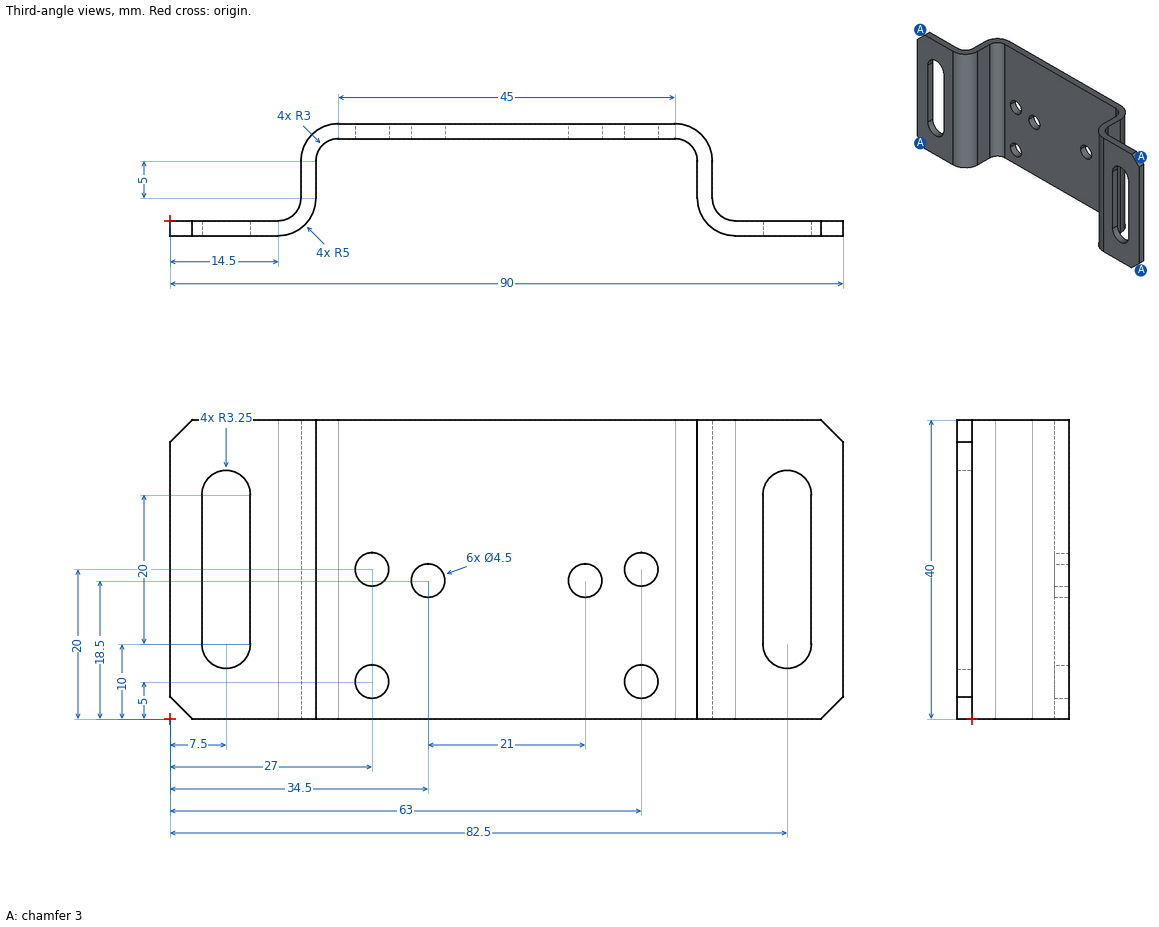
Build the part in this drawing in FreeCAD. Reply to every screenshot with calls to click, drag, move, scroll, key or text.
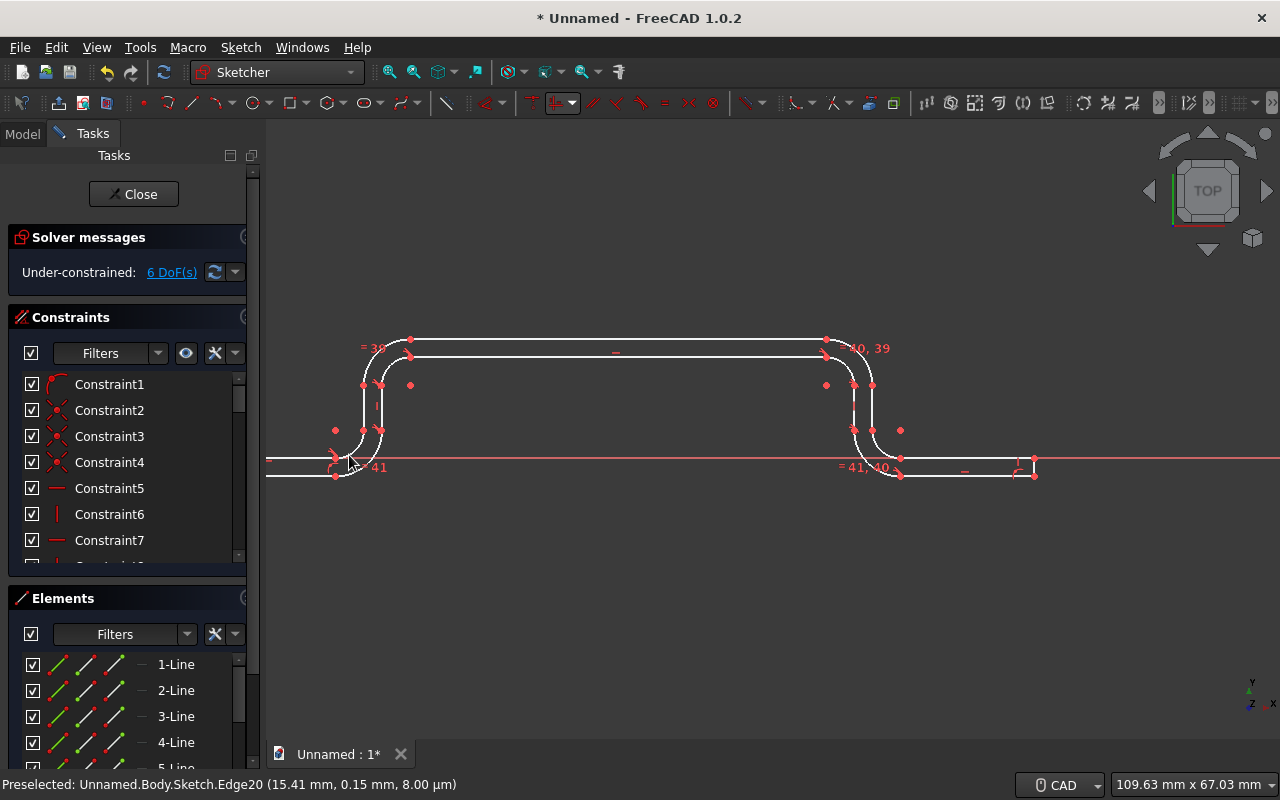
key(d)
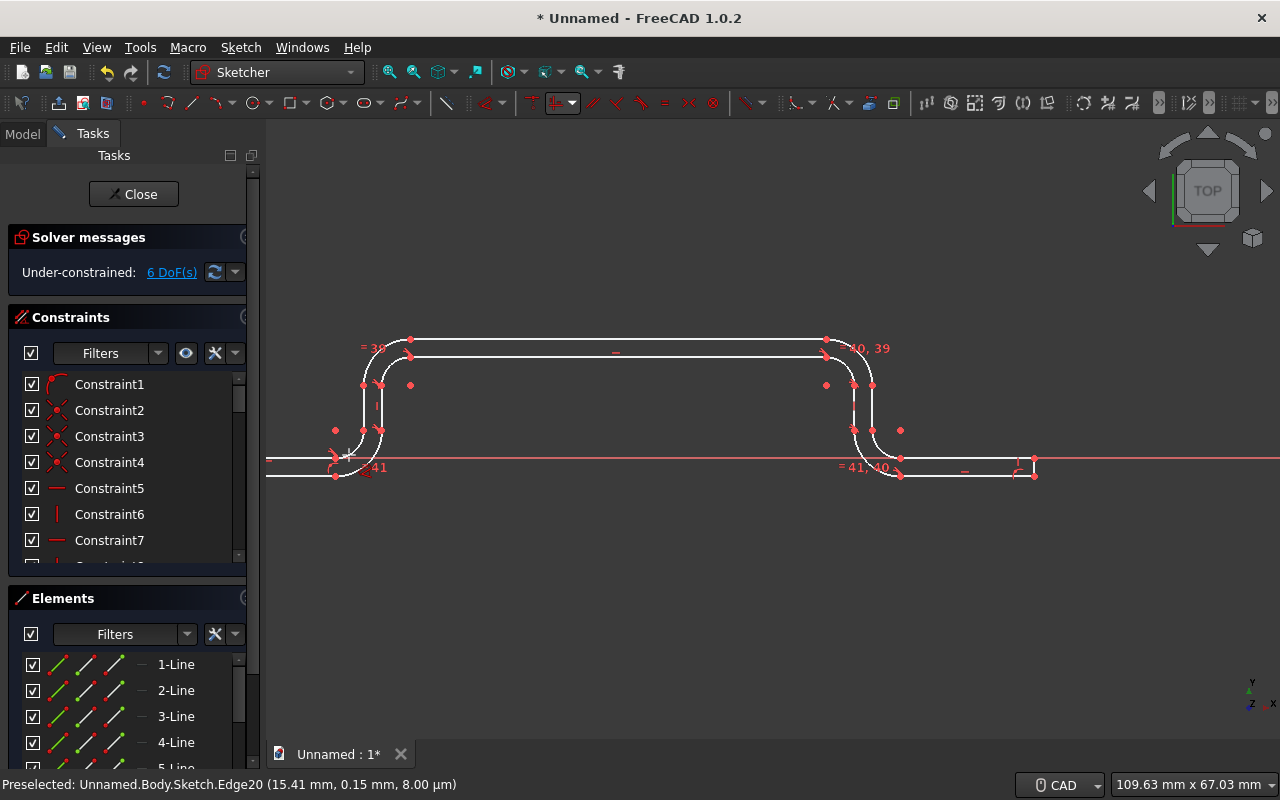
click(357, 471)
click(372, 499)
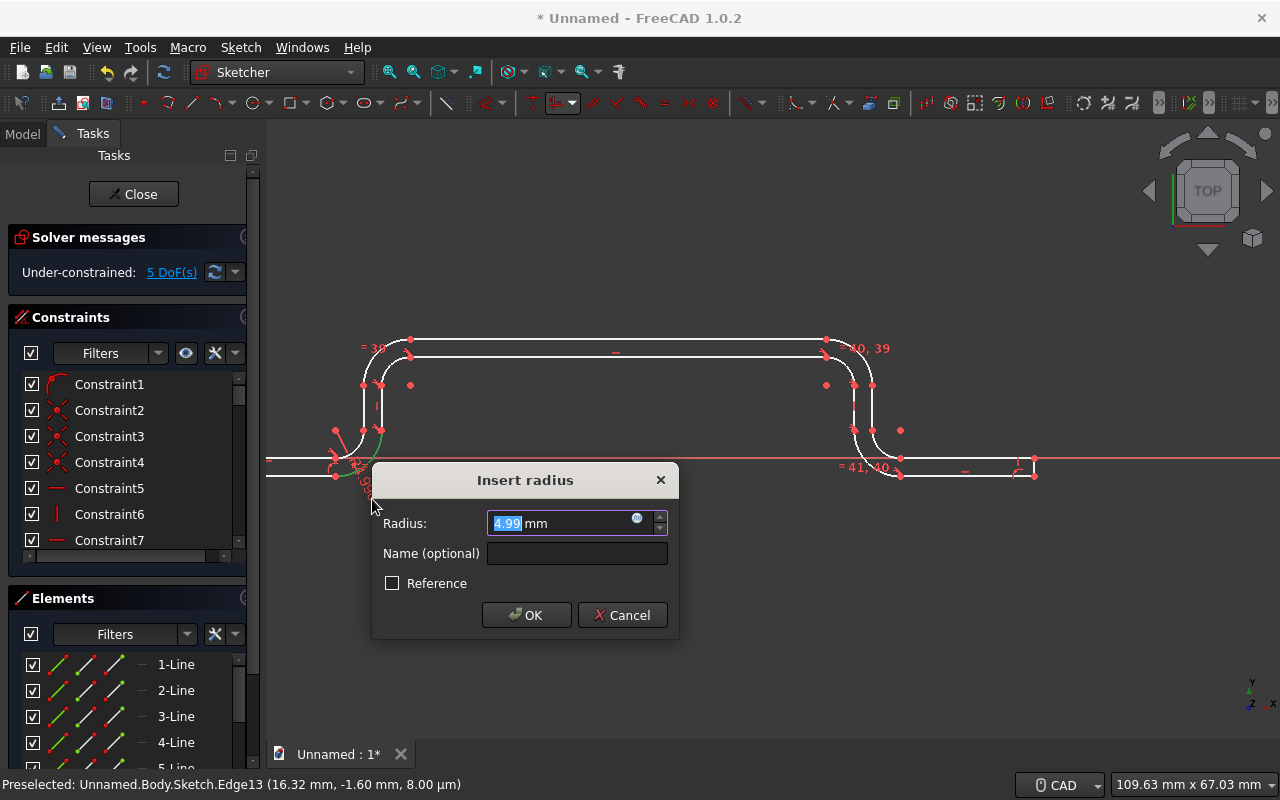
text(5)
key(Return)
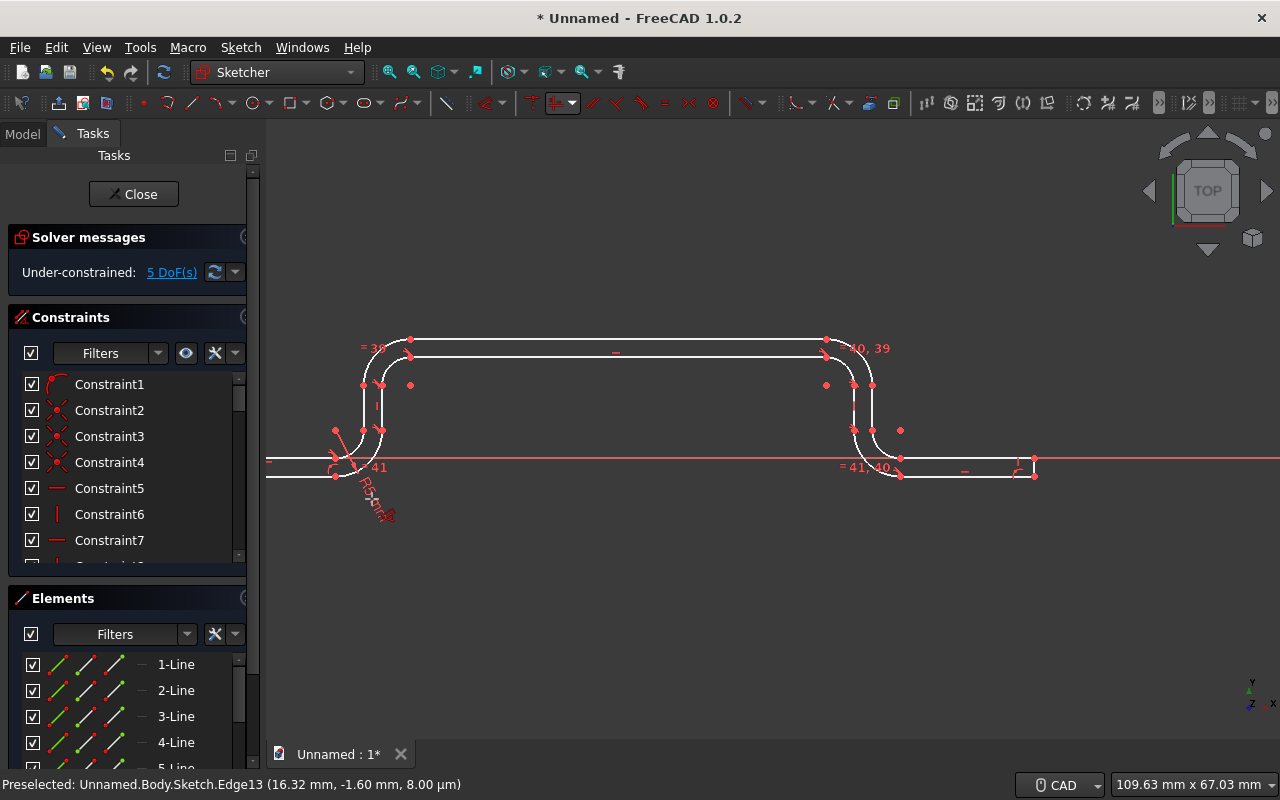
scroll(397, 361, up, 2)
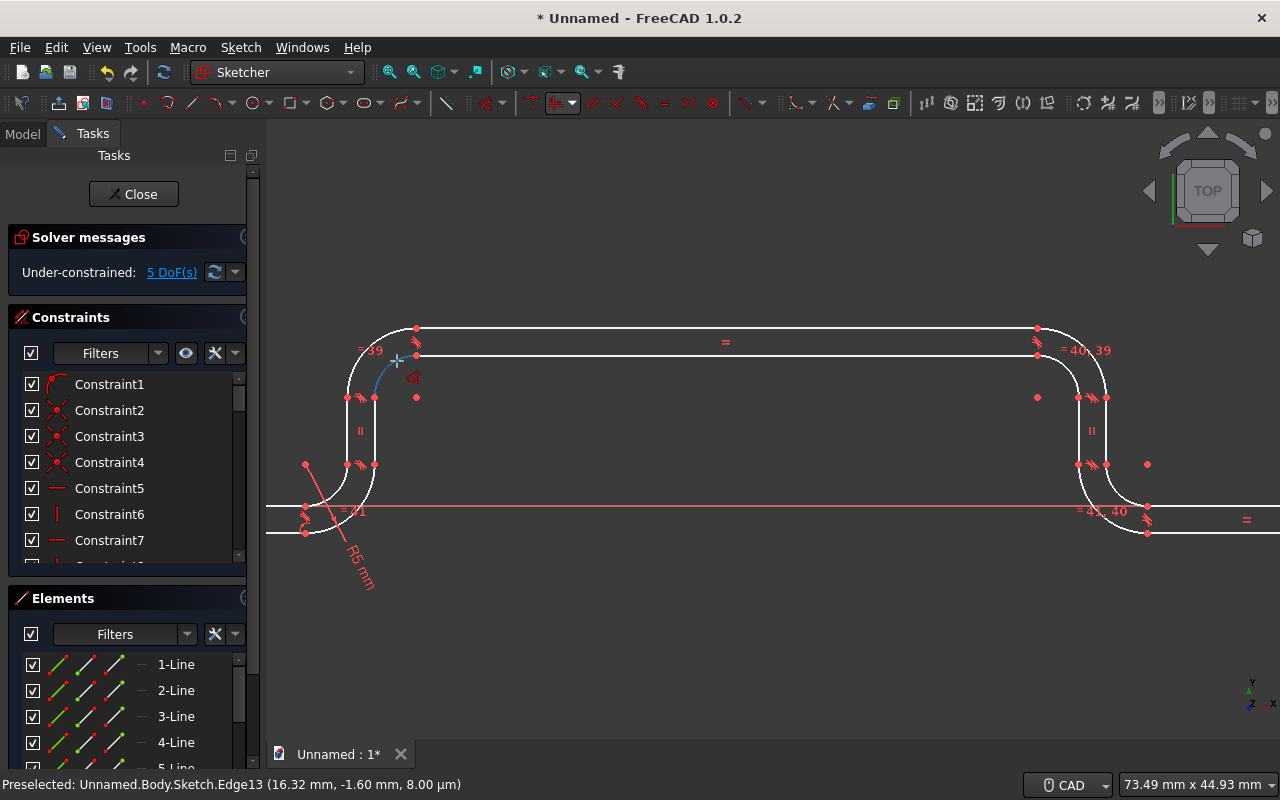
click(398, 360)
click(449, 463)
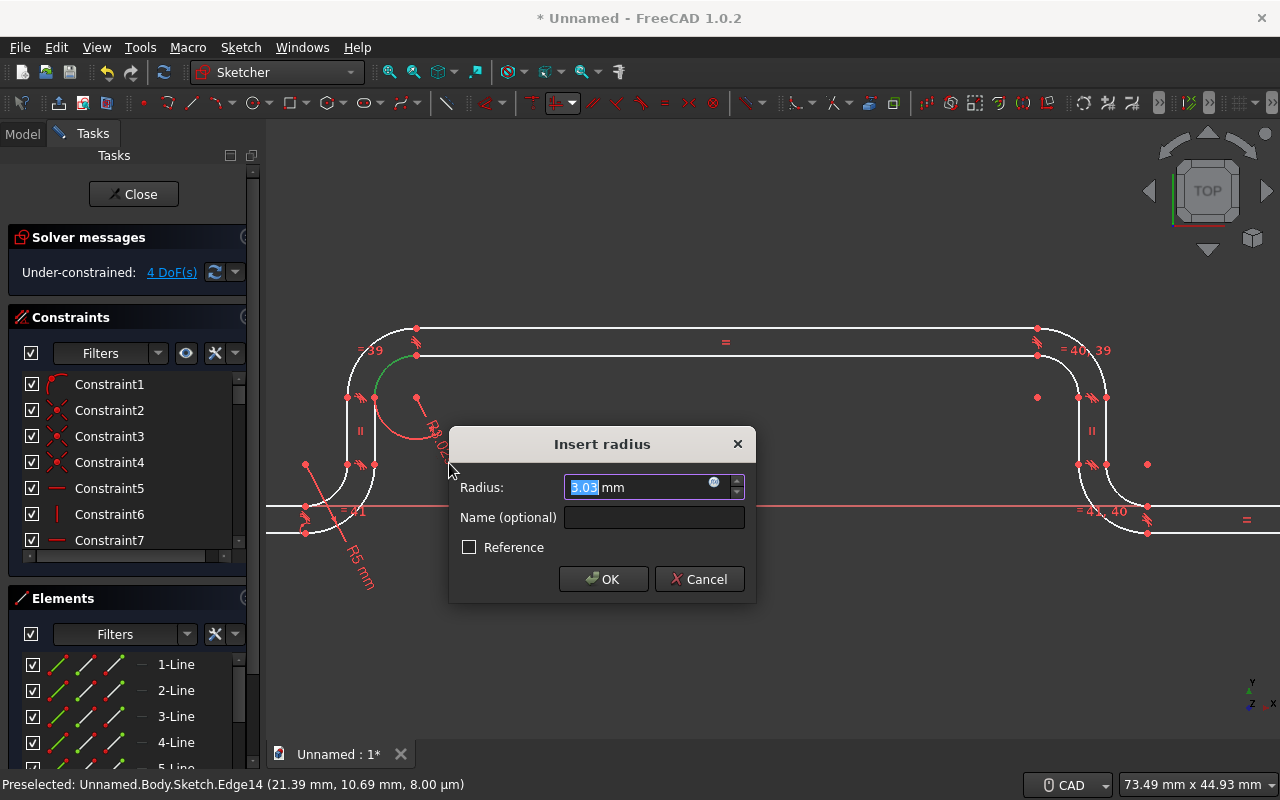
text(3)
key(Return)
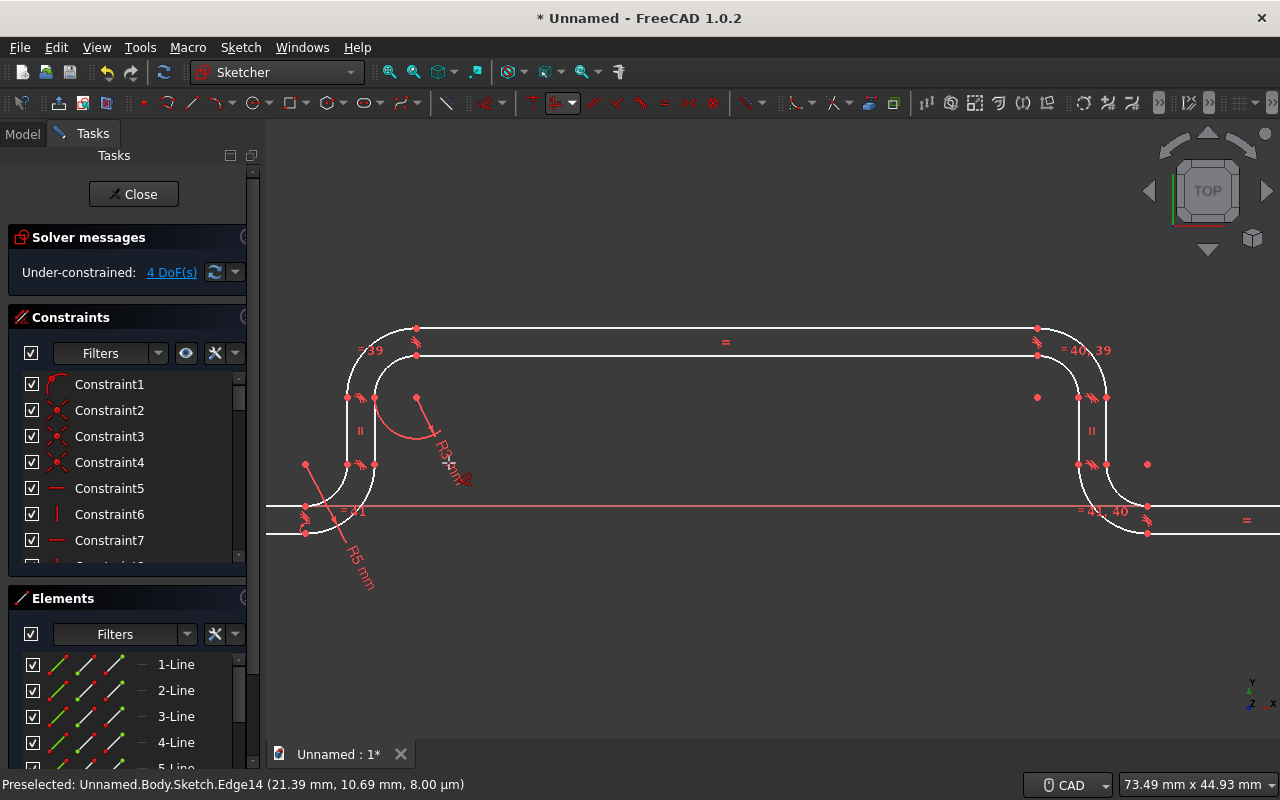
click(375, 444)
click(409, 431)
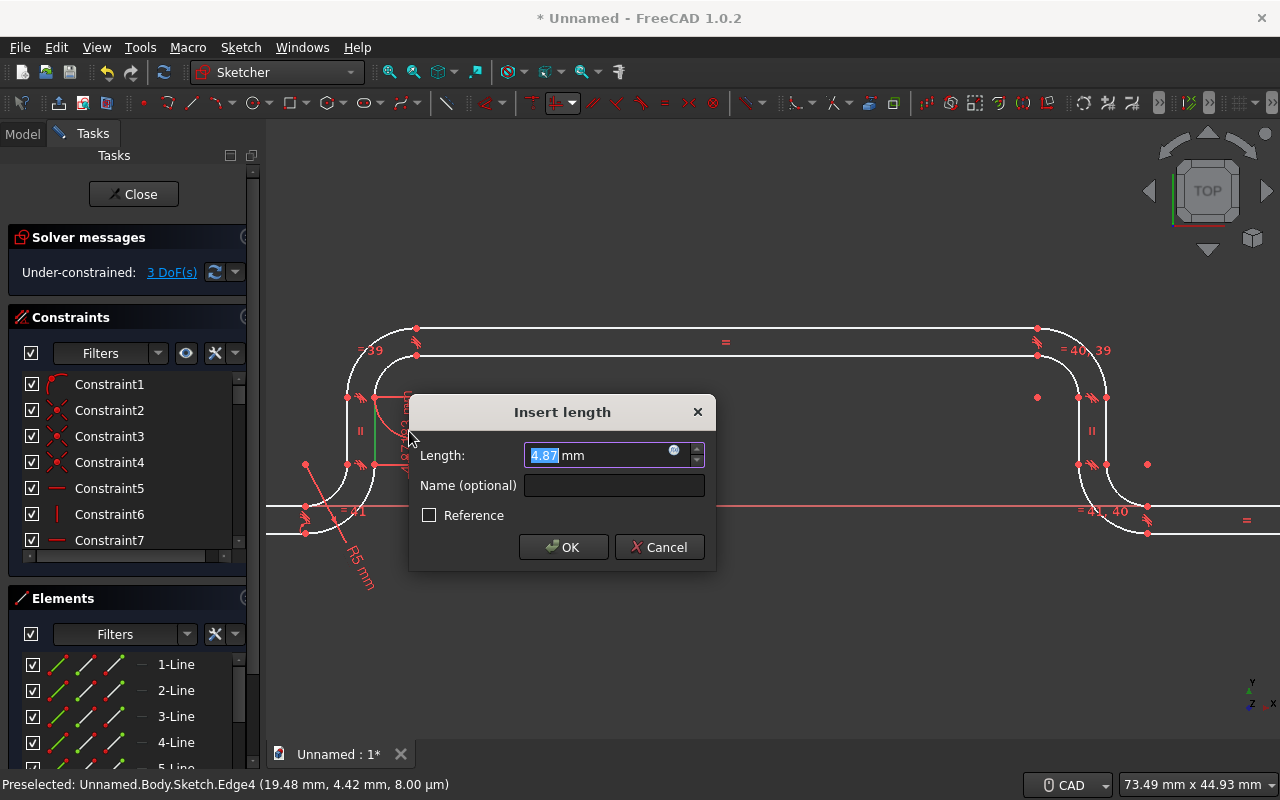
text(5)
key(Return)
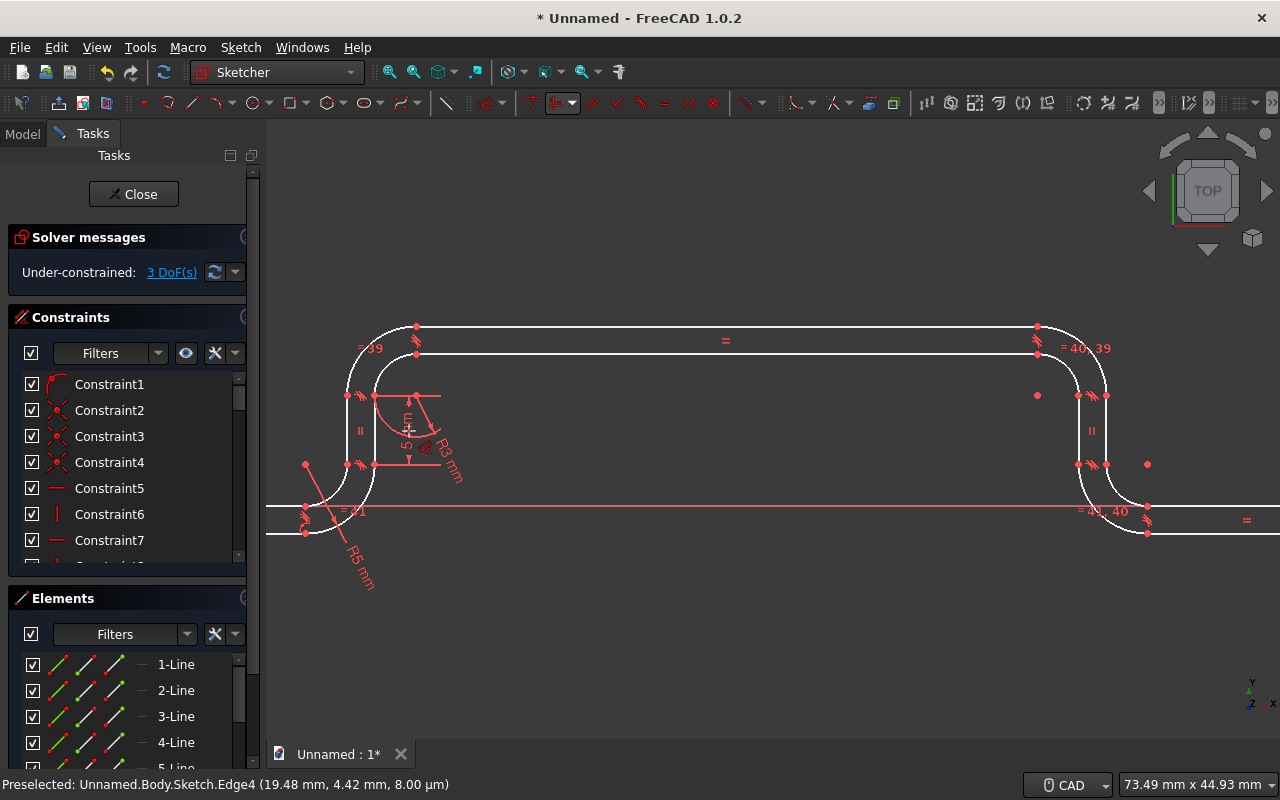
click(602, 354)
click(727, 388)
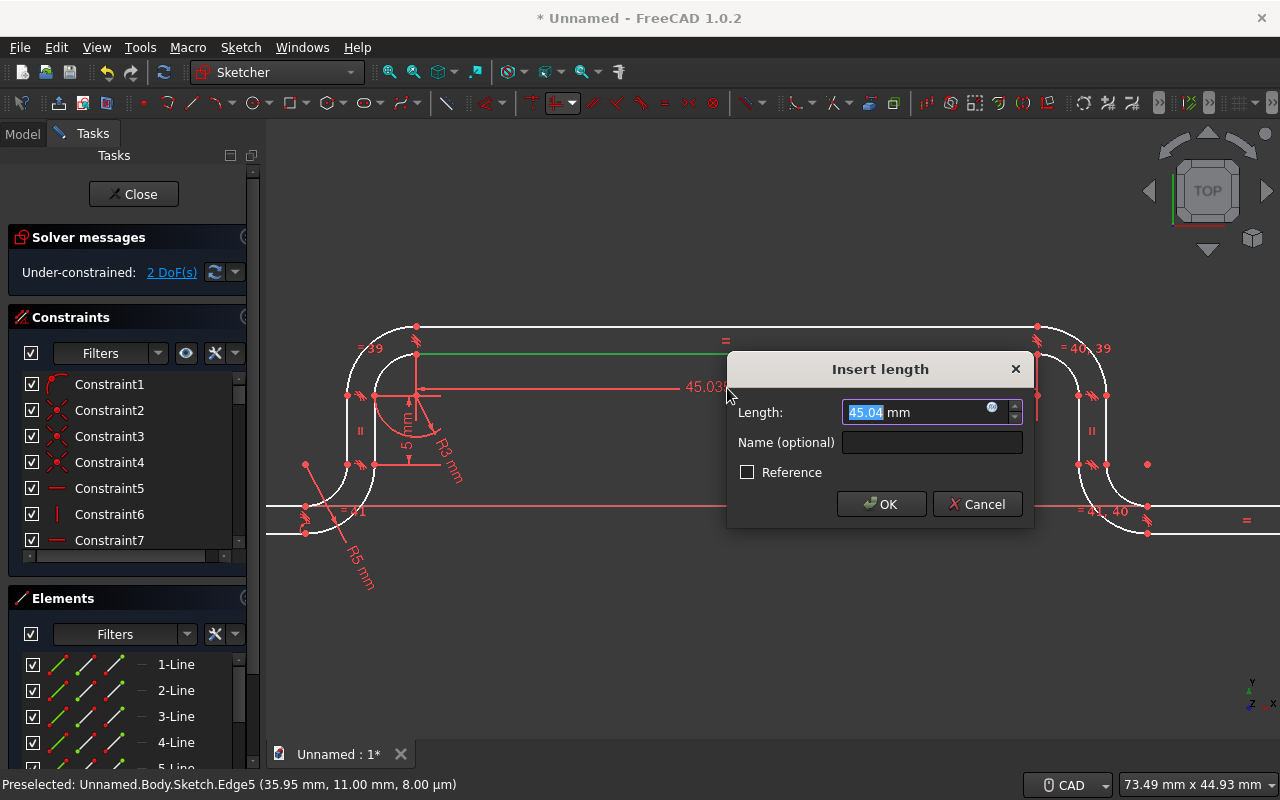
text(45)
key(Return)